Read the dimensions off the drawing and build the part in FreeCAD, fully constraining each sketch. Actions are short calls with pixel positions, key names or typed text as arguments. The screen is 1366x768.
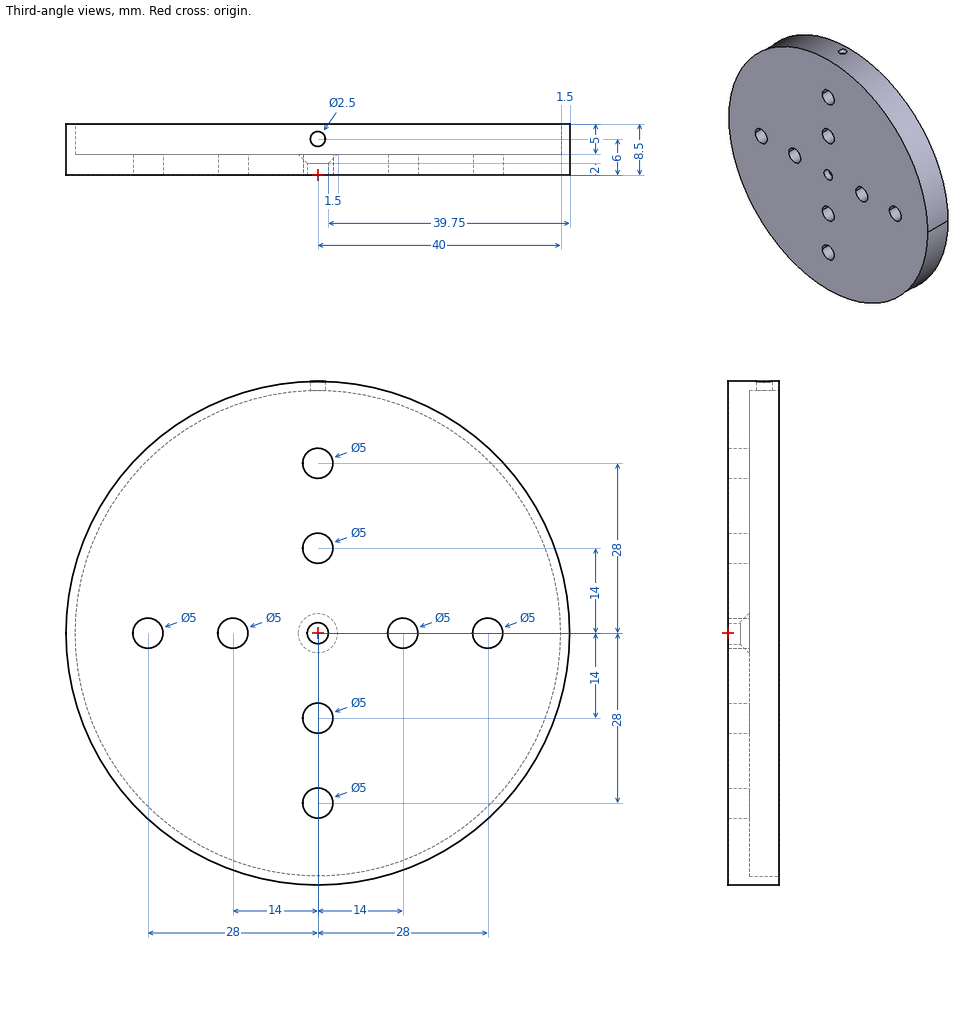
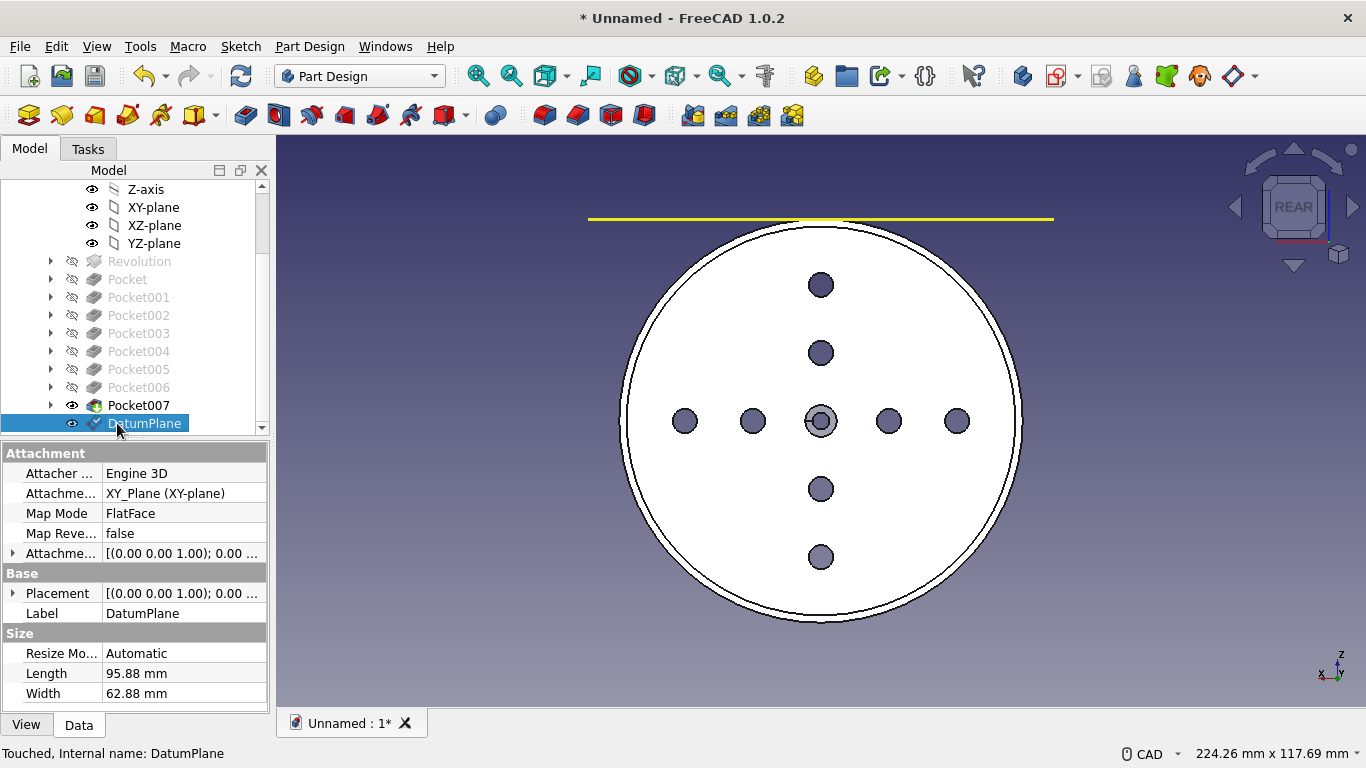
click(1056, 76)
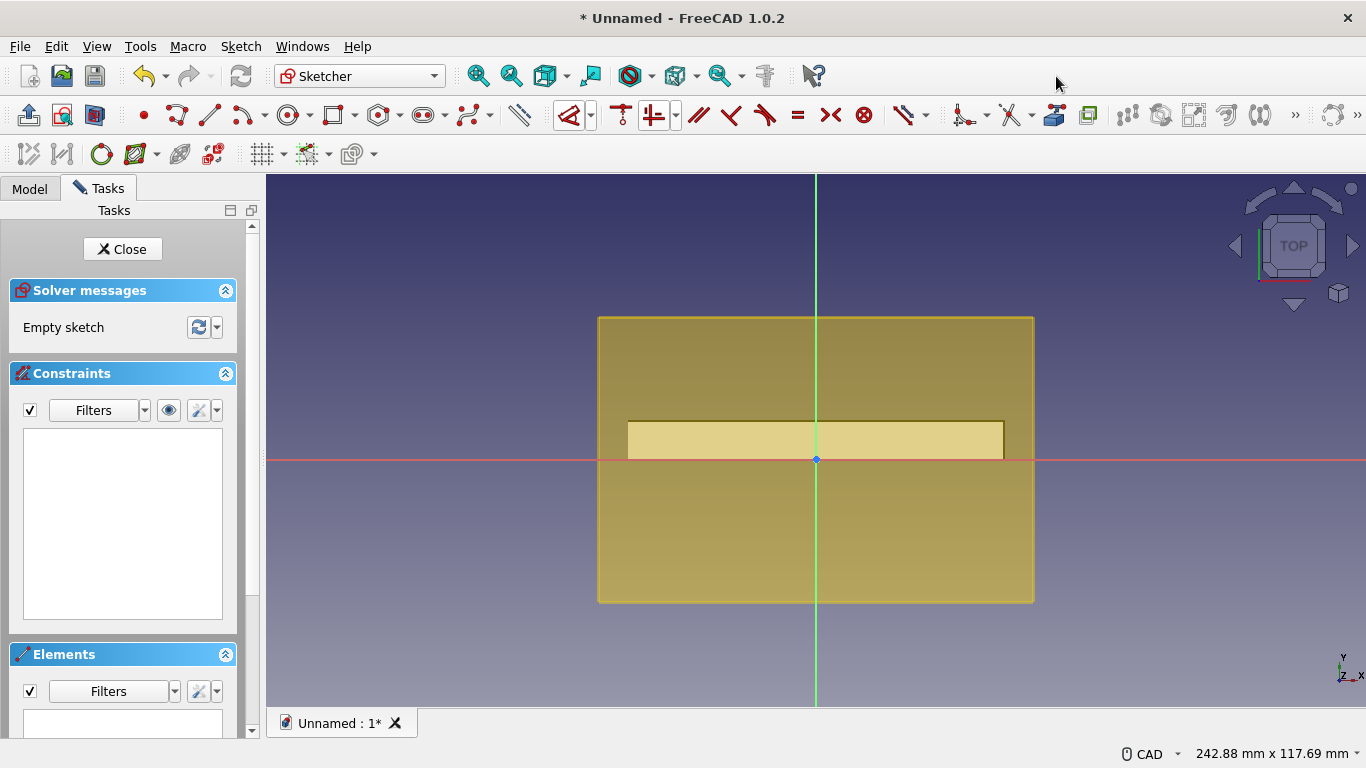
scroll(820, 432, up, 15)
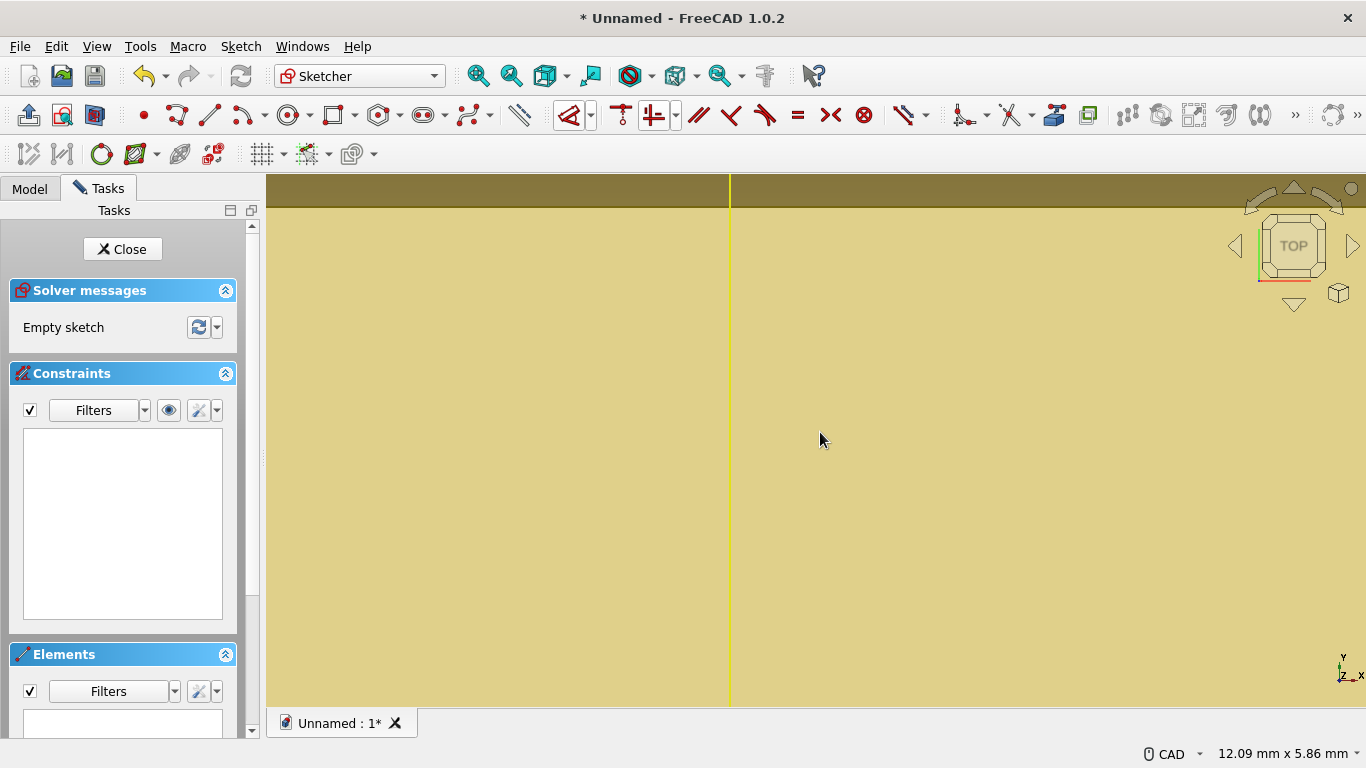
scroll(695, 422, up, 2)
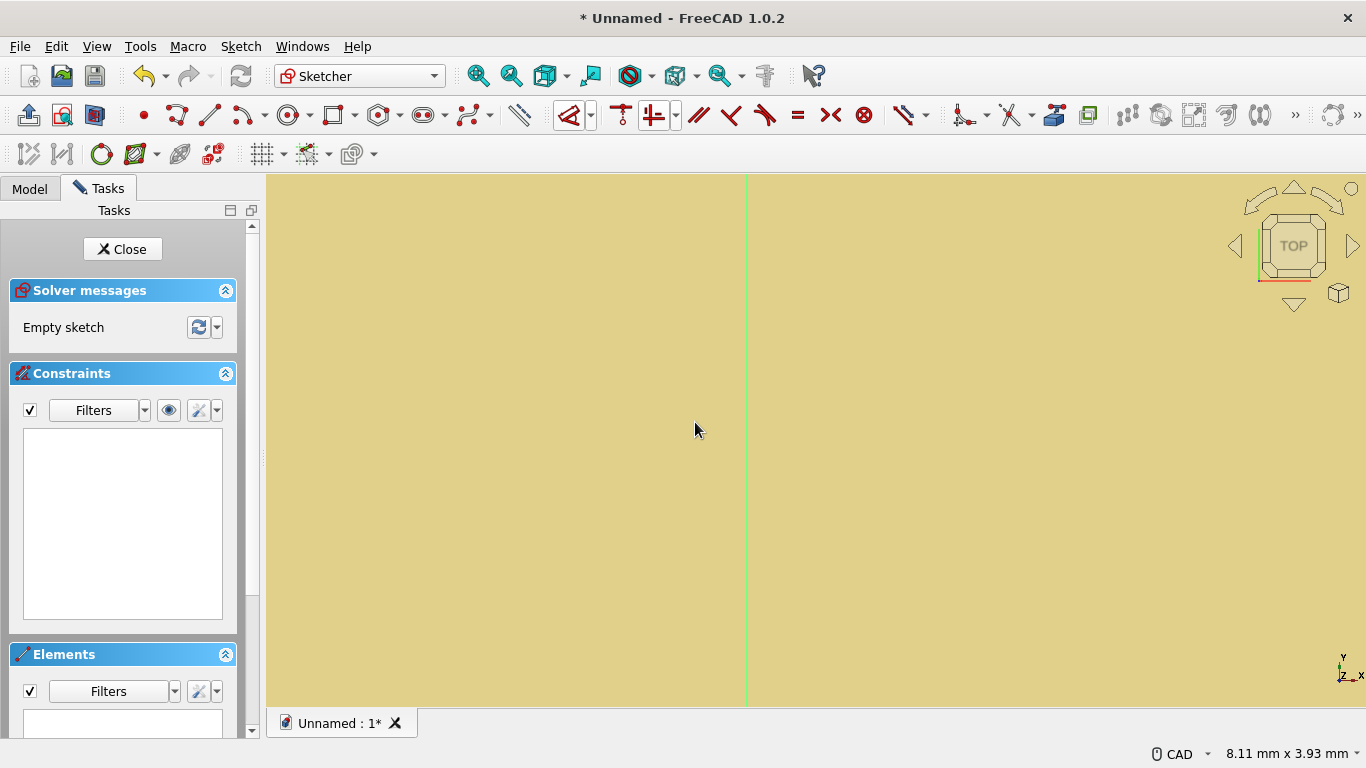
click(288, 116)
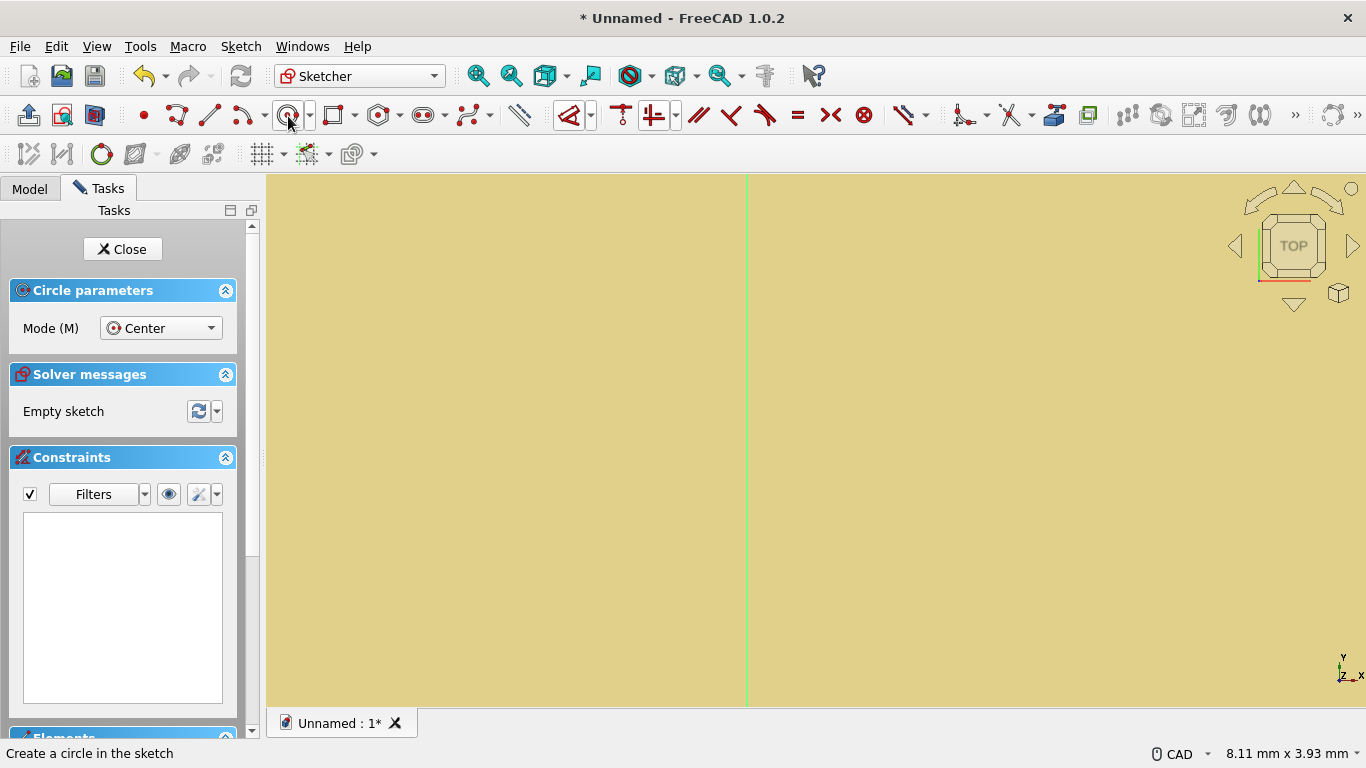
click(747, 440)
click(867, 320)
key(Escape)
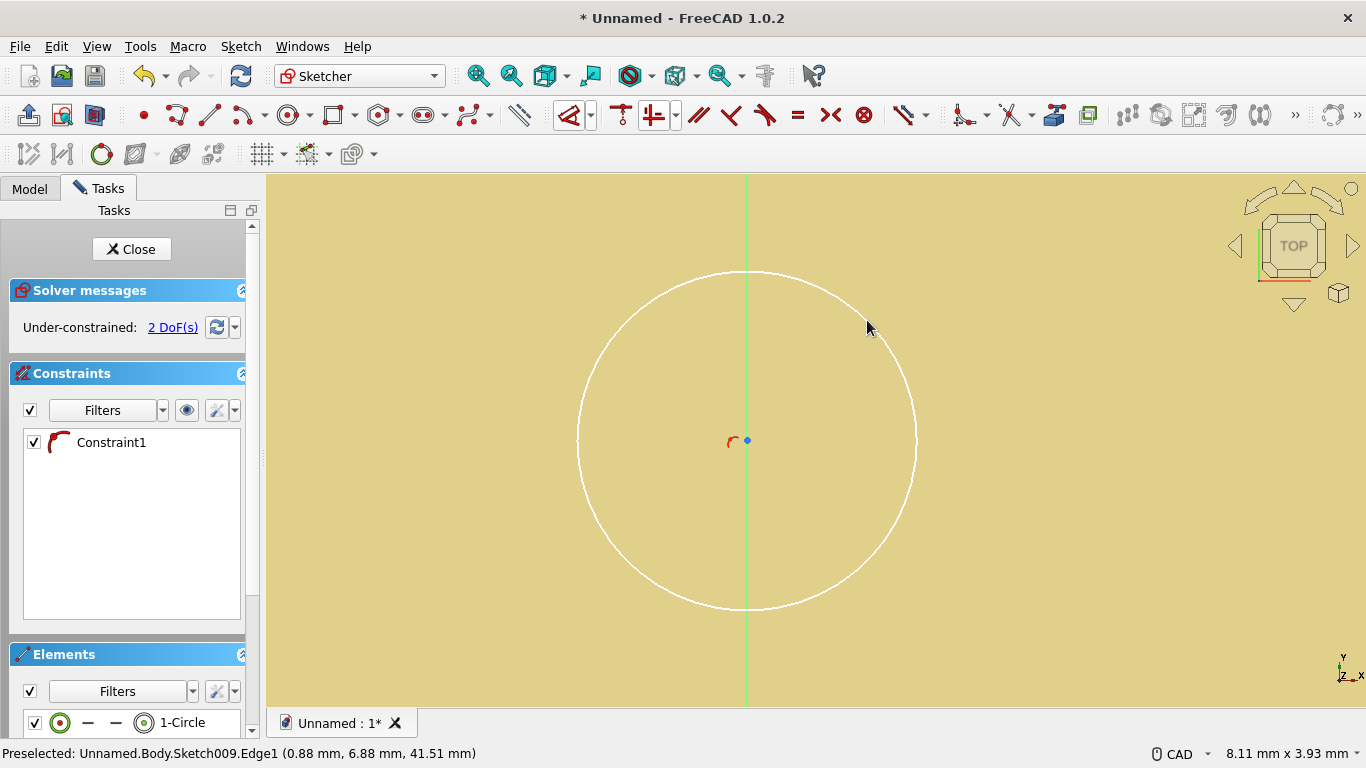
click(867, 321)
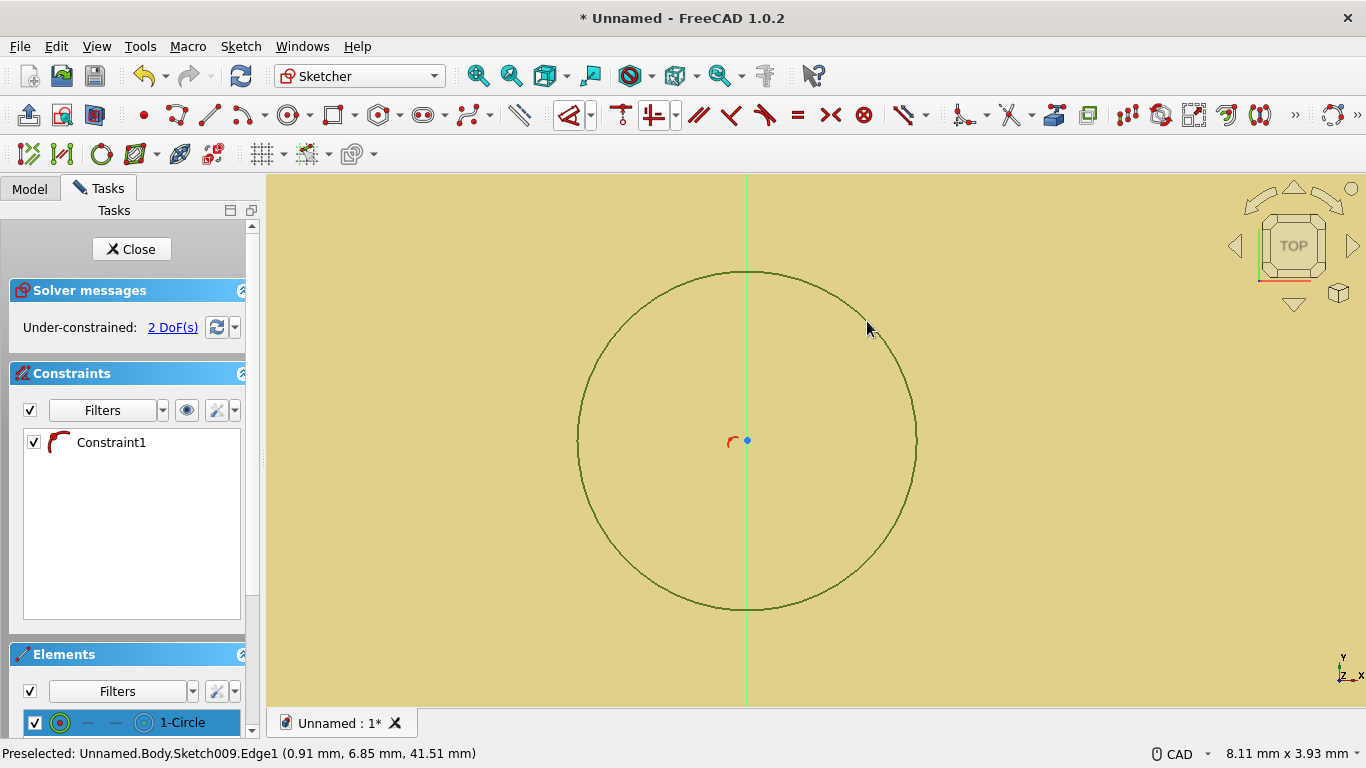
key(k)
key(o)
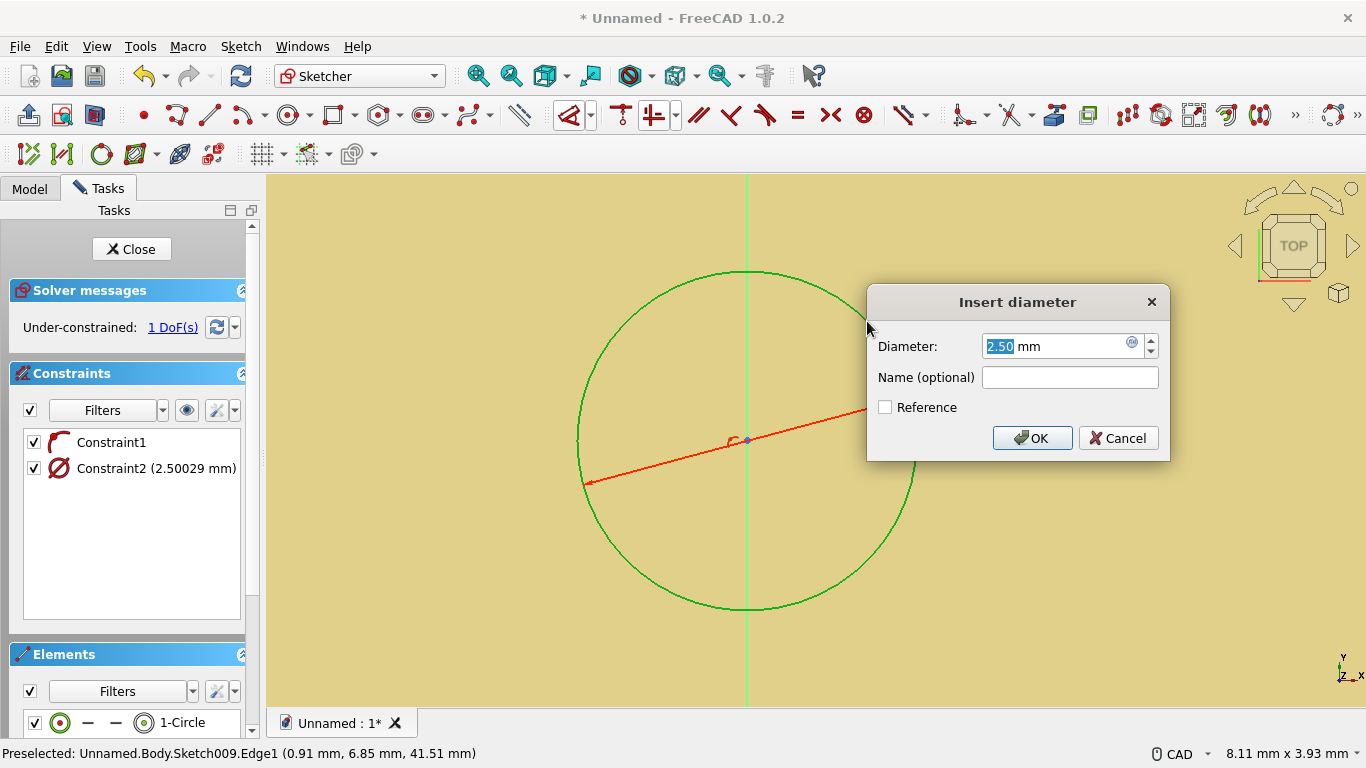
text(2.5)
key(Return)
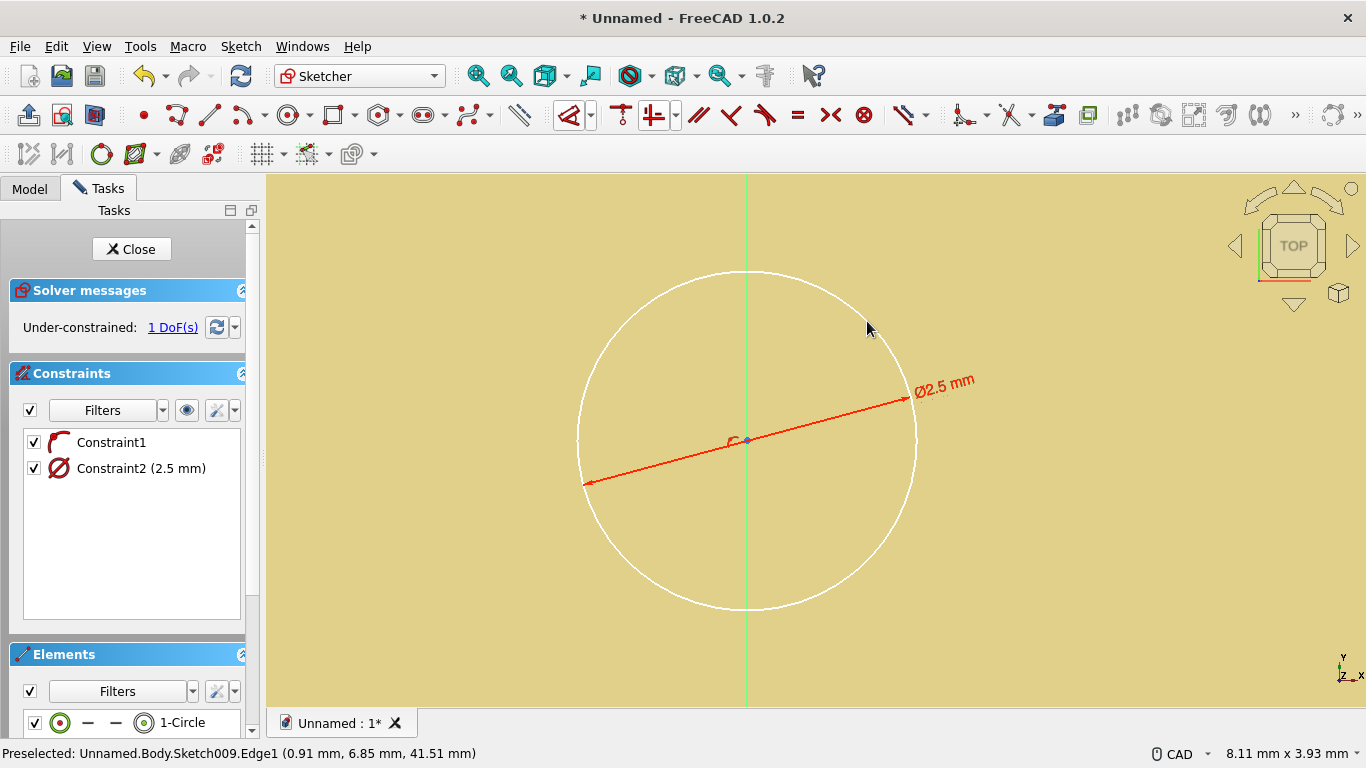
click(747, 441)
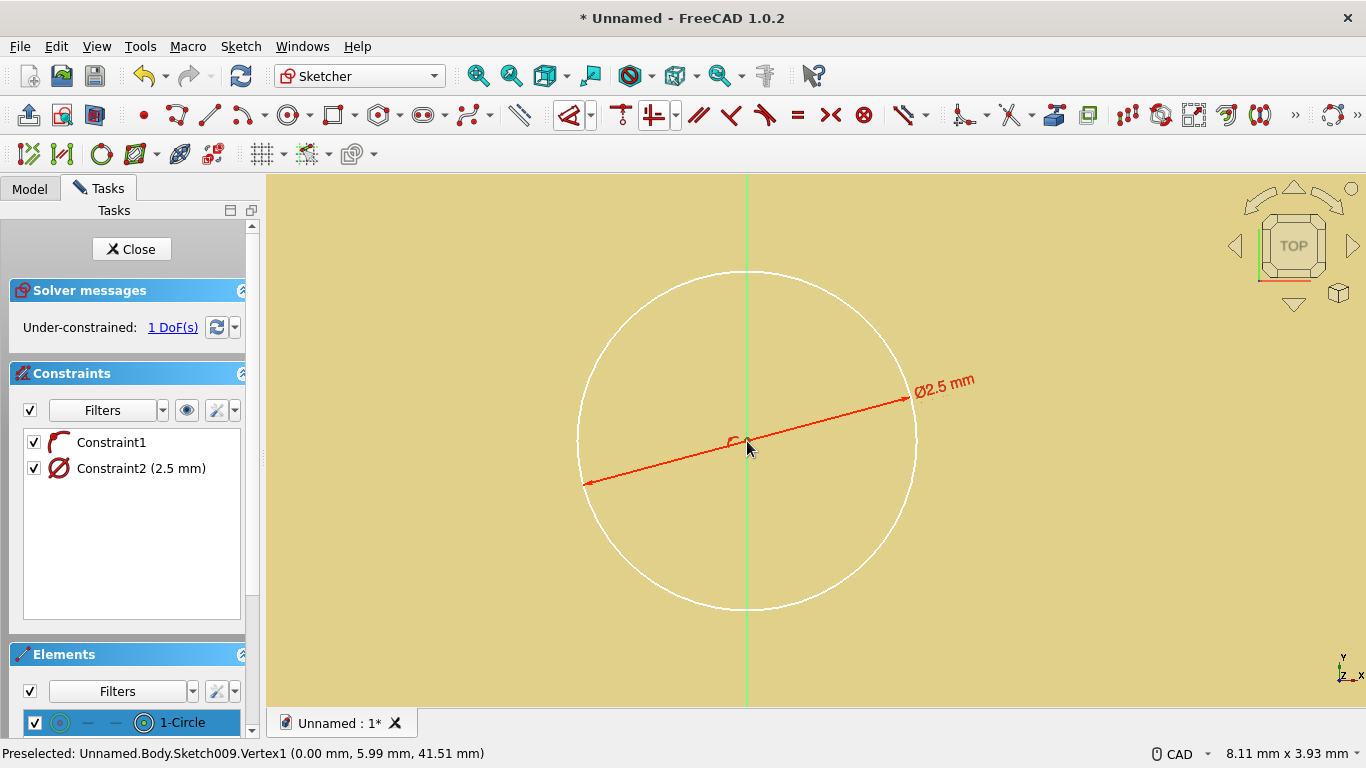
key(i)